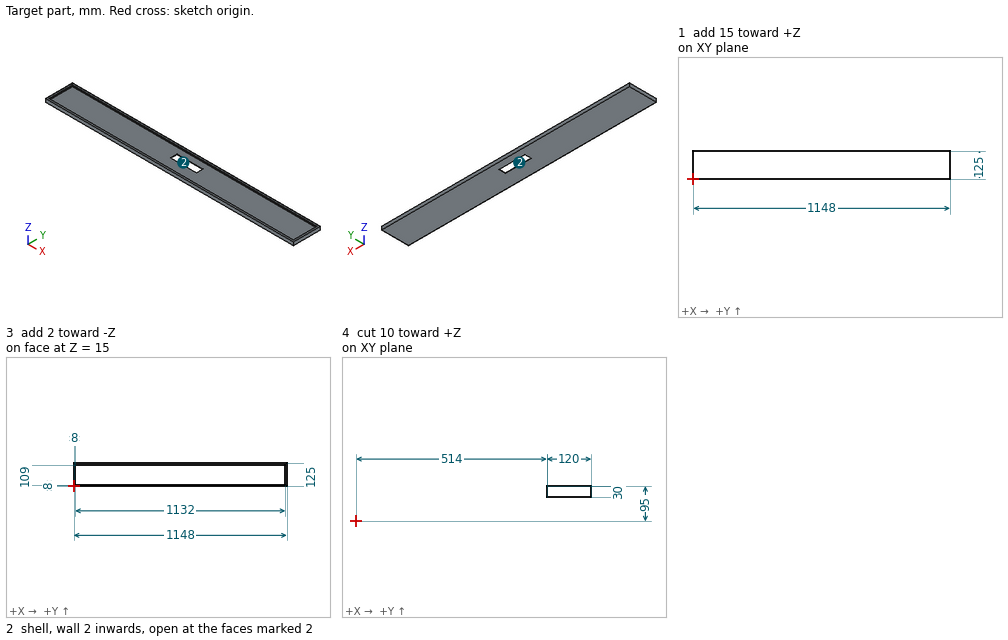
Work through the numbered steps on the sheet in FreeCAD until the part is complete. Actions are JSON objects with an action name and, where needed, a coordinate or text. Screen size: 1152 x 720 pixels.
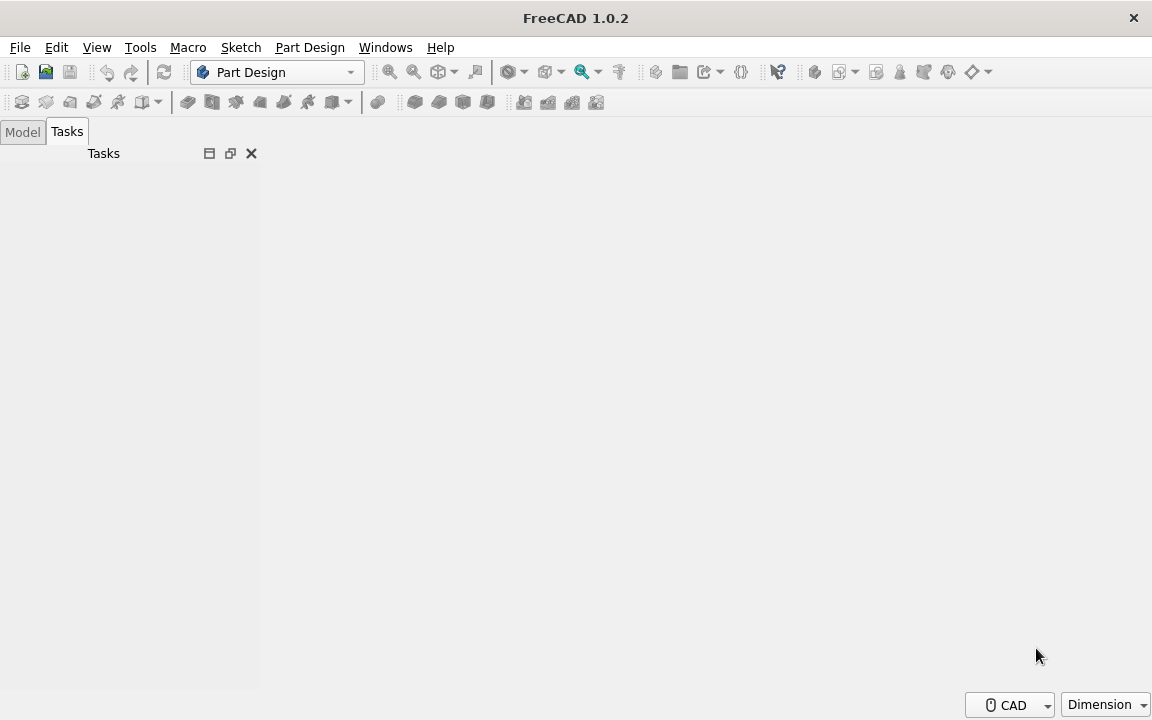
{"action": "left_click", "coordinate": [22, 72]}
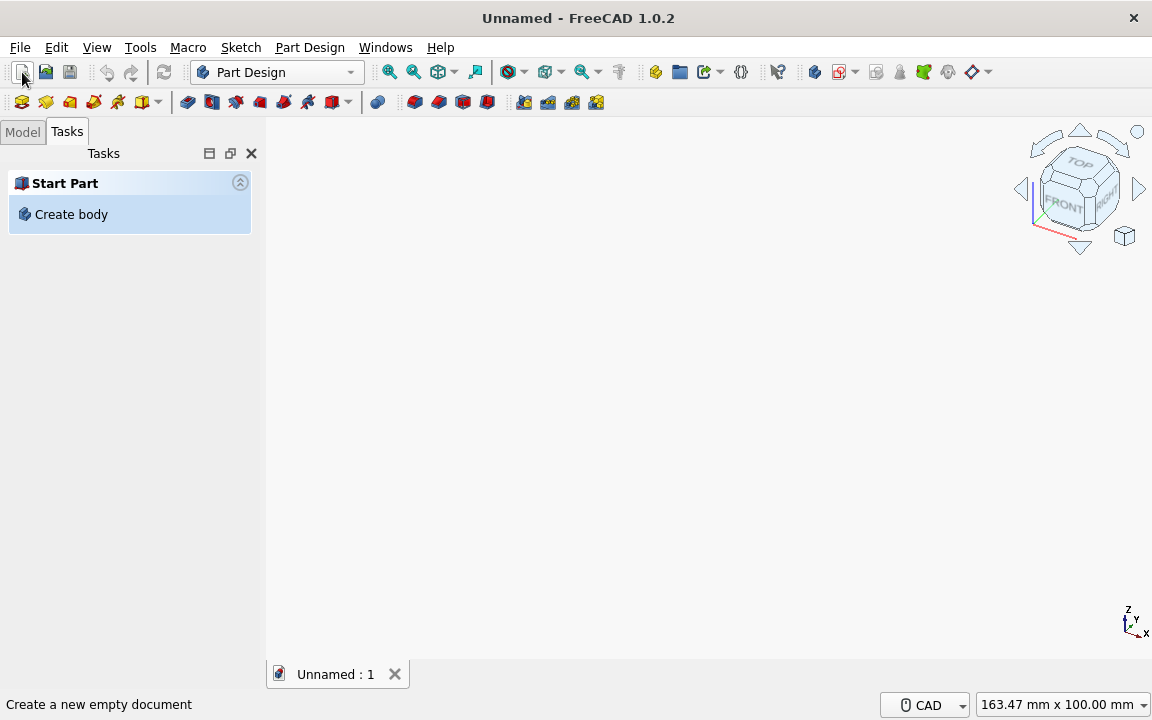
{"action": "left_click", "coordinate": [840, 72]}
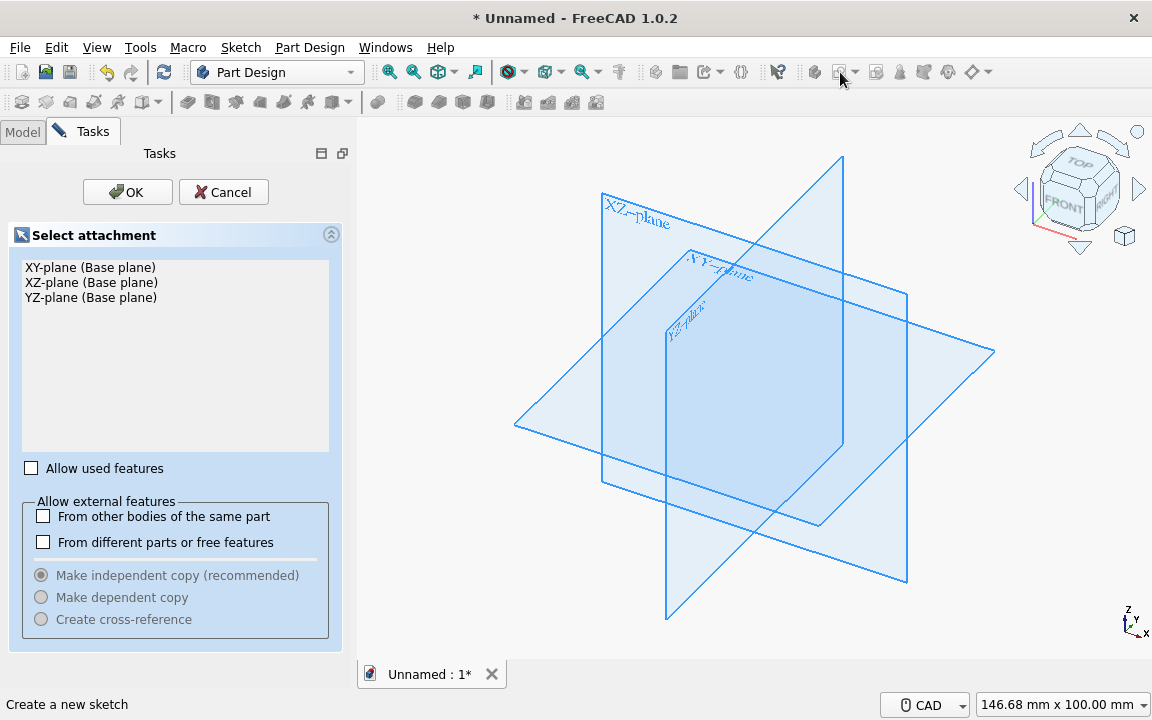
{"action": "left_click", "coordinate": [82, 268]}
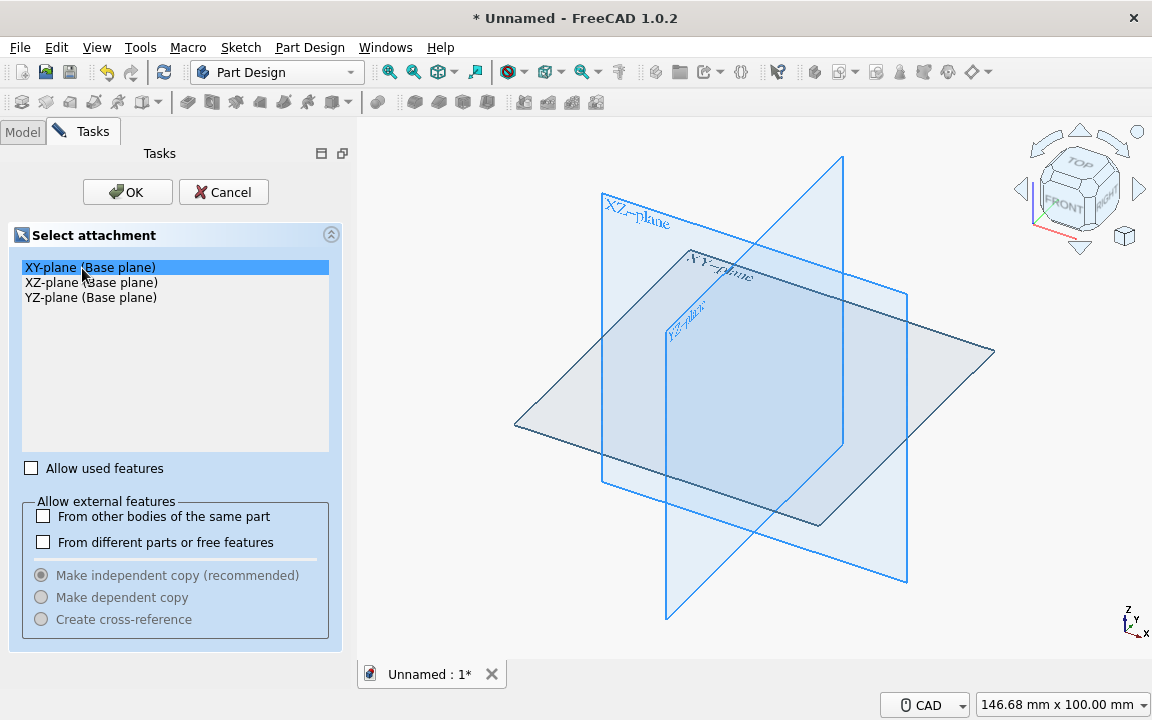
{"action": "left_click", "coordinate": [128, 192]}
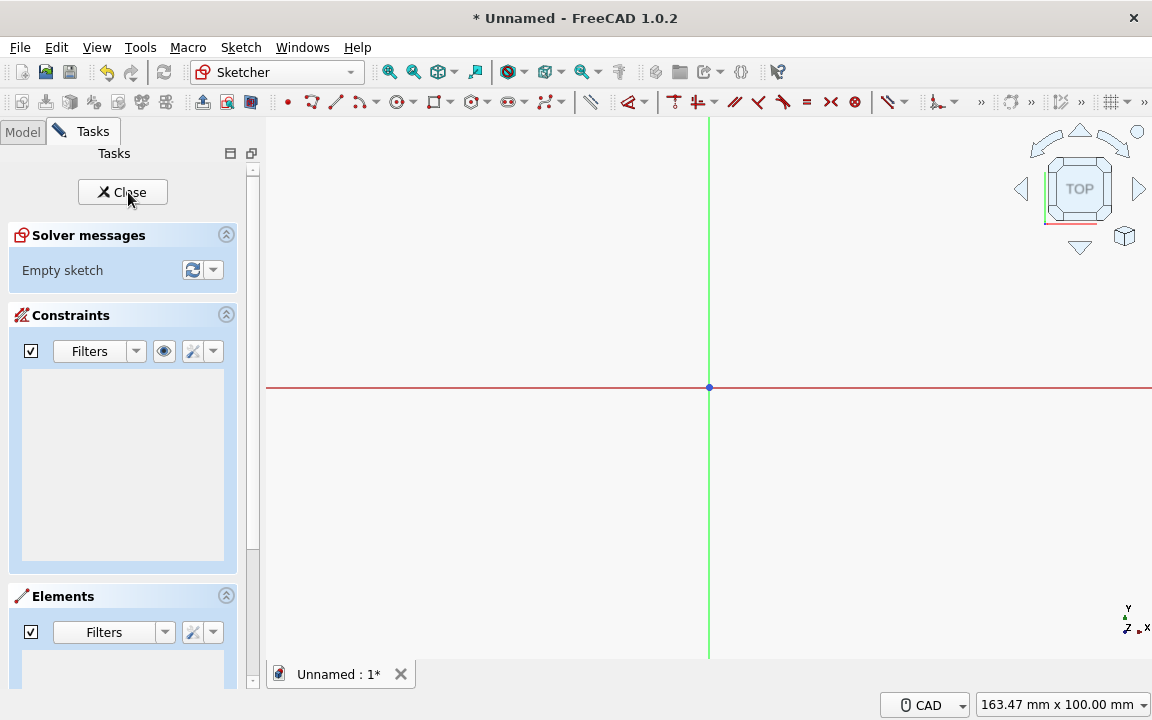
{"action": "scroll", "coordinate": [385, 415], "scroll_direction": "down", "scroll_amount": 13}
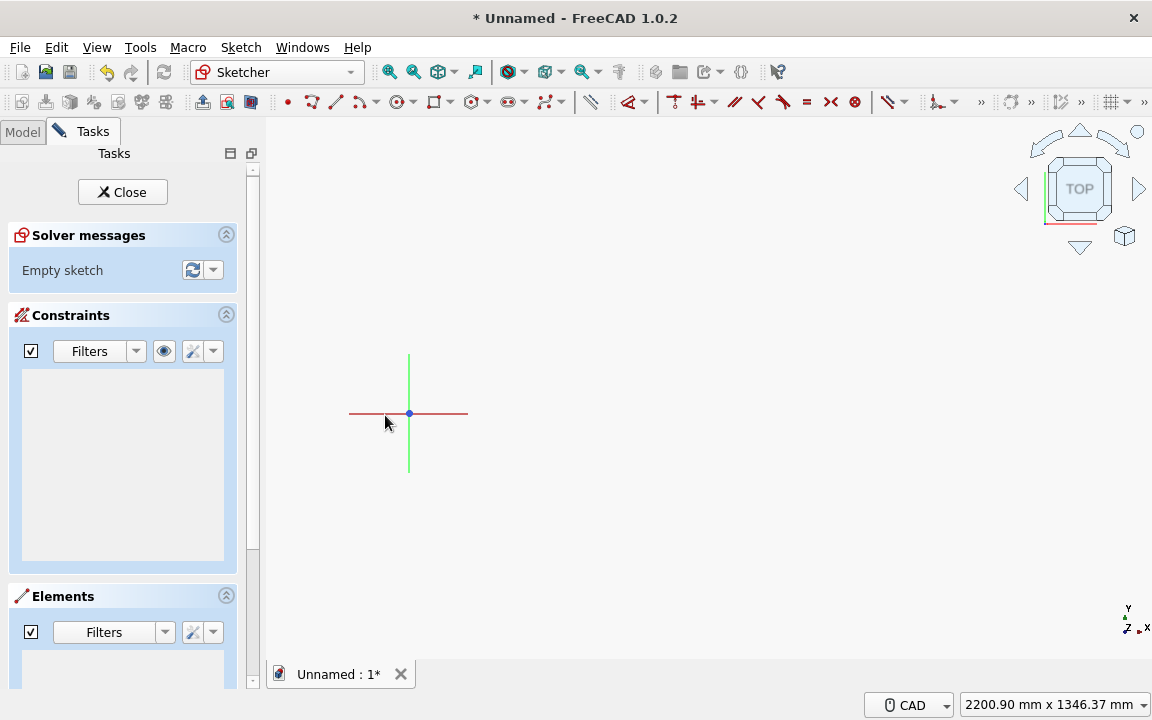
{"action": "left_click", "coordinate": [434, 102]}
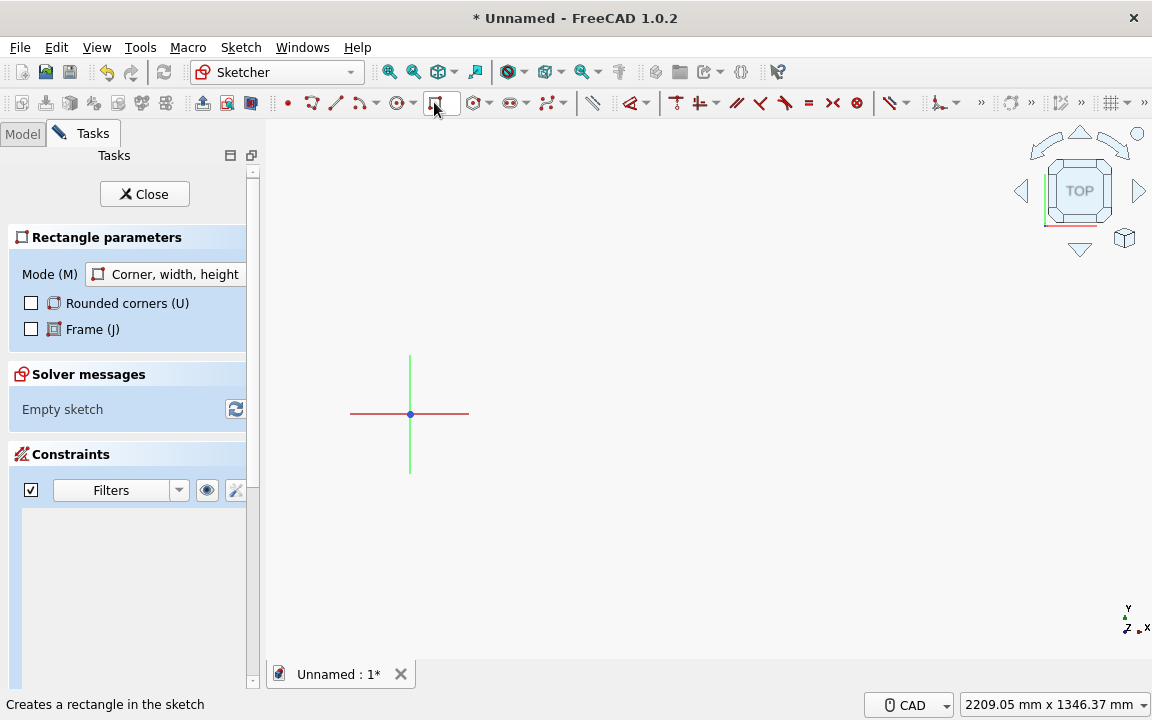
{"action": "left_click", "coordinate": [410, 414]}
{"action": "mouse_move", "coordinate": [871, 364]}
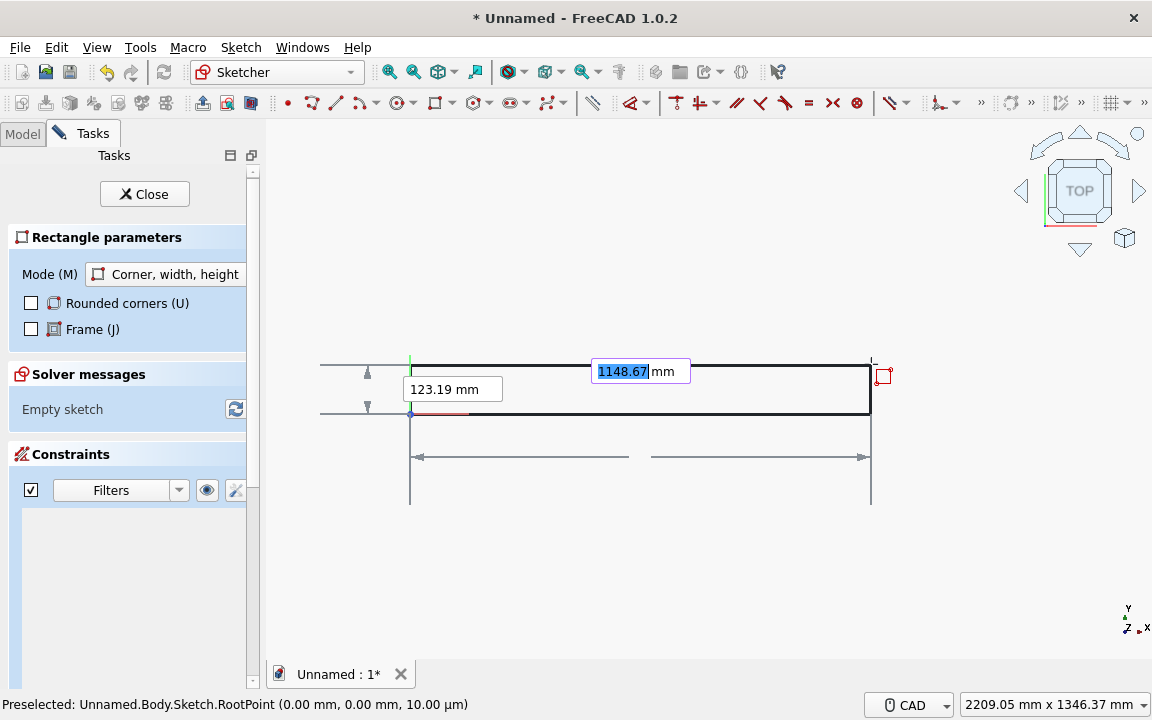
{"action": "type", "text": "1148"}
{"action": "key", "text": "Tab"}
{"action": "type", "text": "125"}
{"action": "key", "text": "Return"}
{"action": "key", "text": "Escape"}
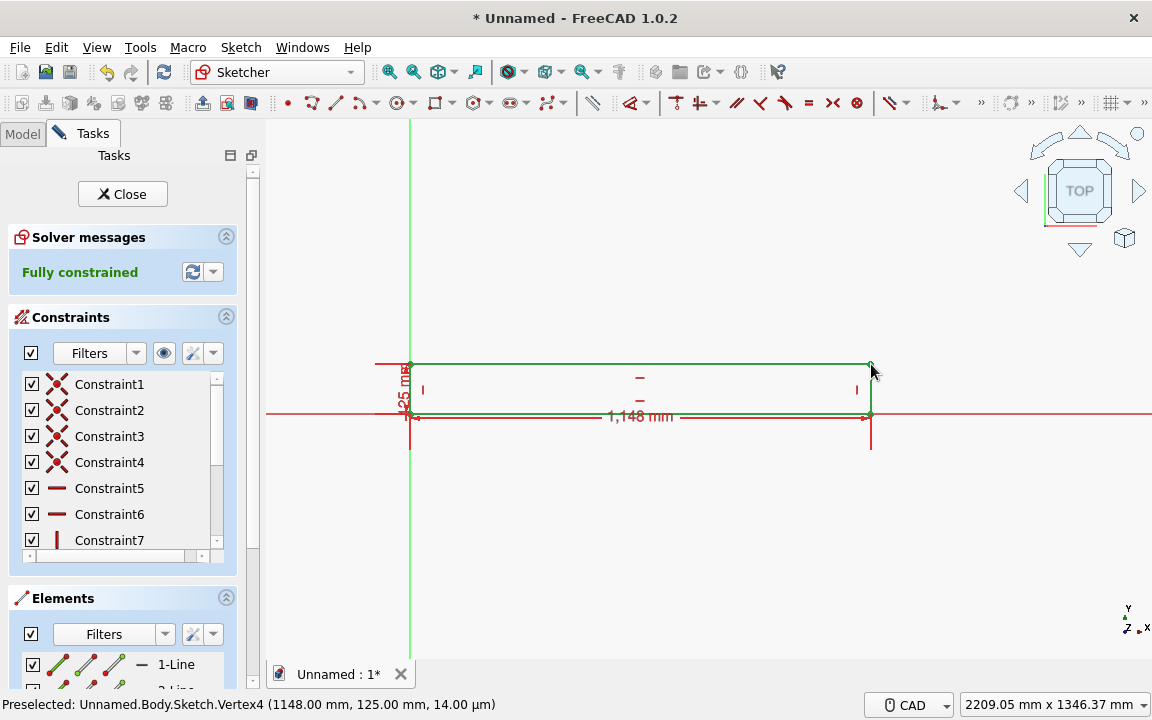
{"action": "left_click", "coordinate": [123, 194]}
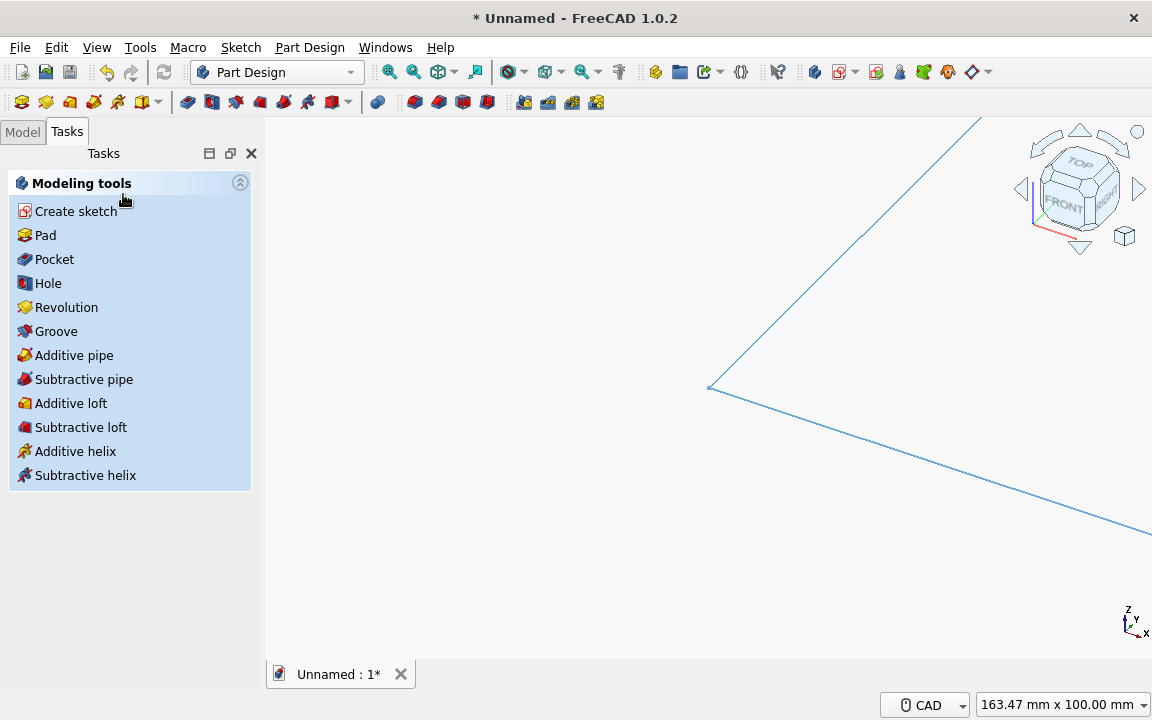
{"action": "left_click", "coordinate": [22, 102]}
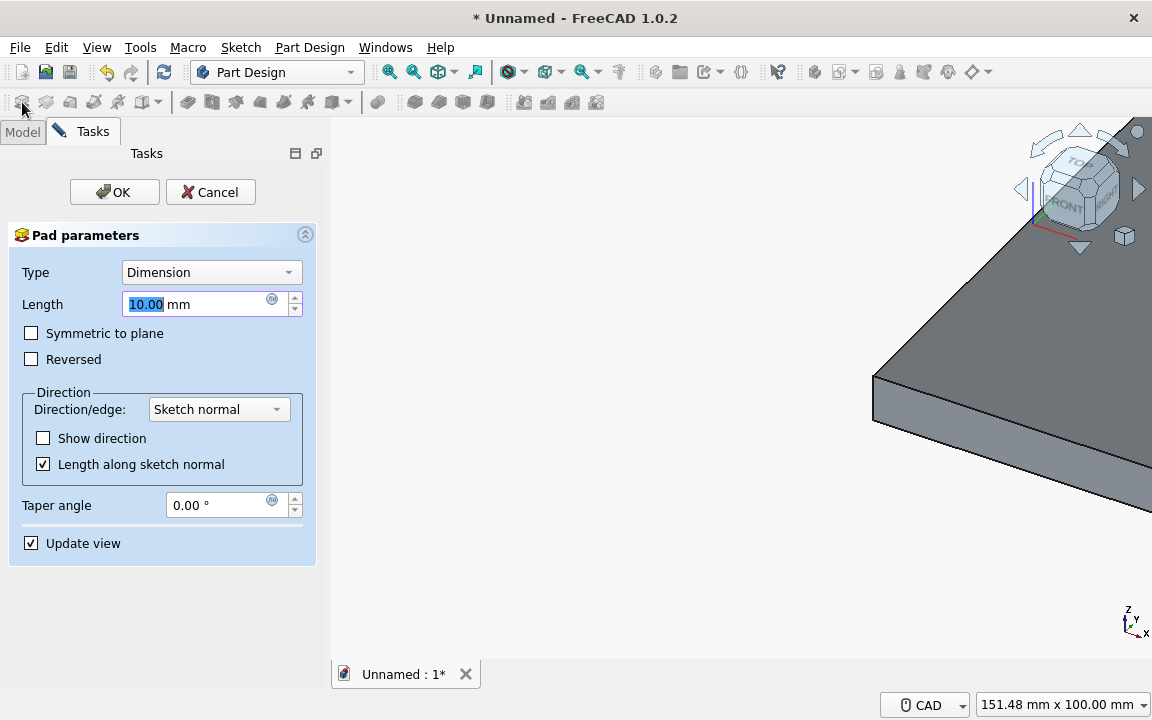
{"action": "type", "text": "15"}
{"action": "key", "text": "Tab"}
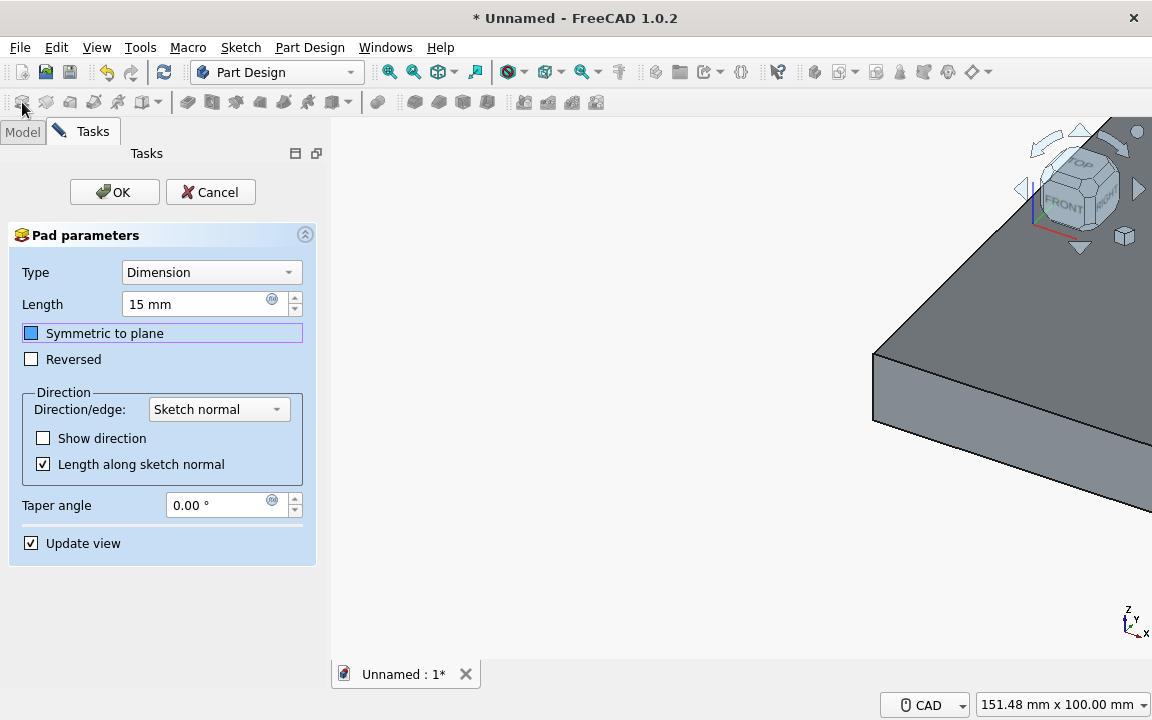
{"action": "left_click", "coordinate": [115, 192]}